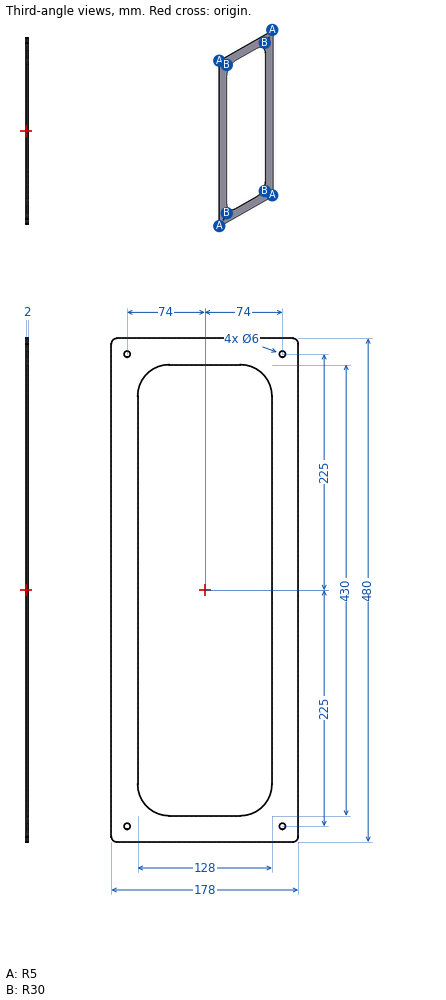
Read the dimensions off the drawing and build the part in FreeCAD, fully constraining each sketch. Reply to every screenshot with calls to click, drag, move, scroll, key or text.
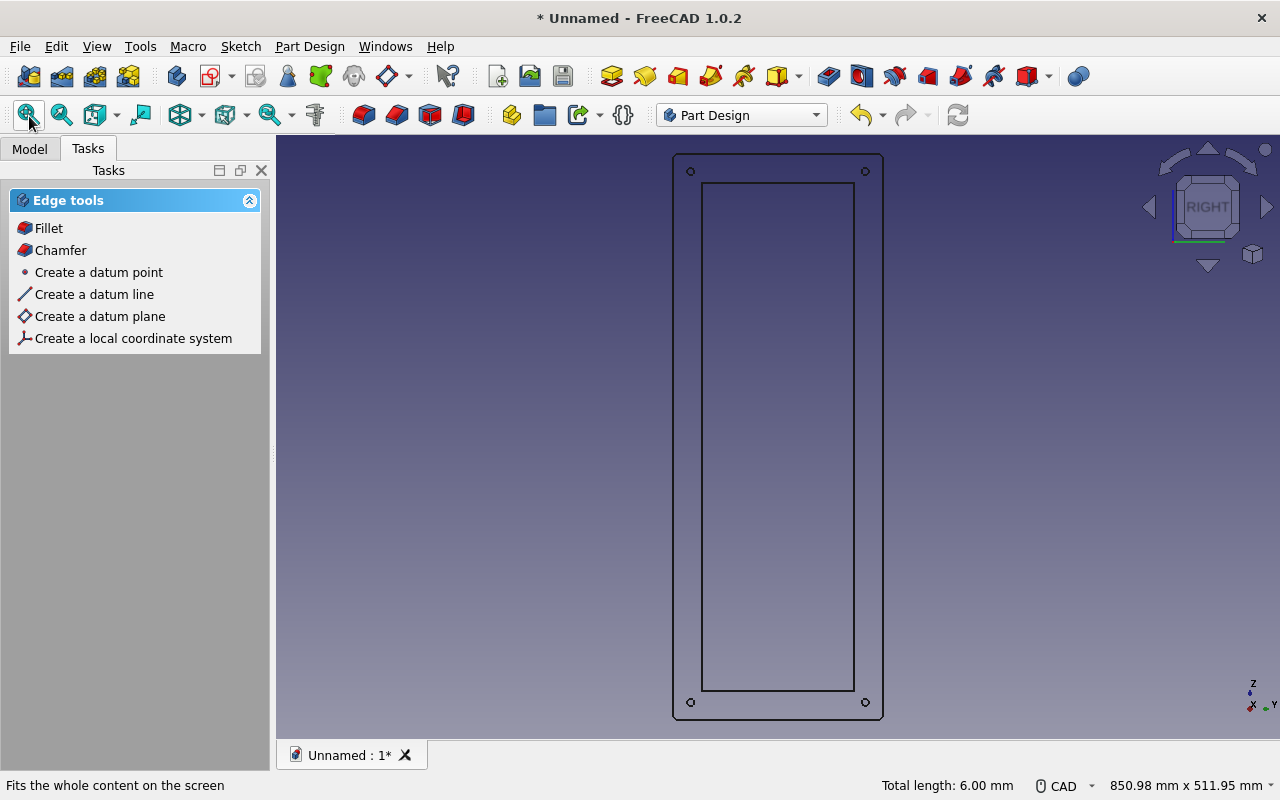
scroll(854, 690, up, 15)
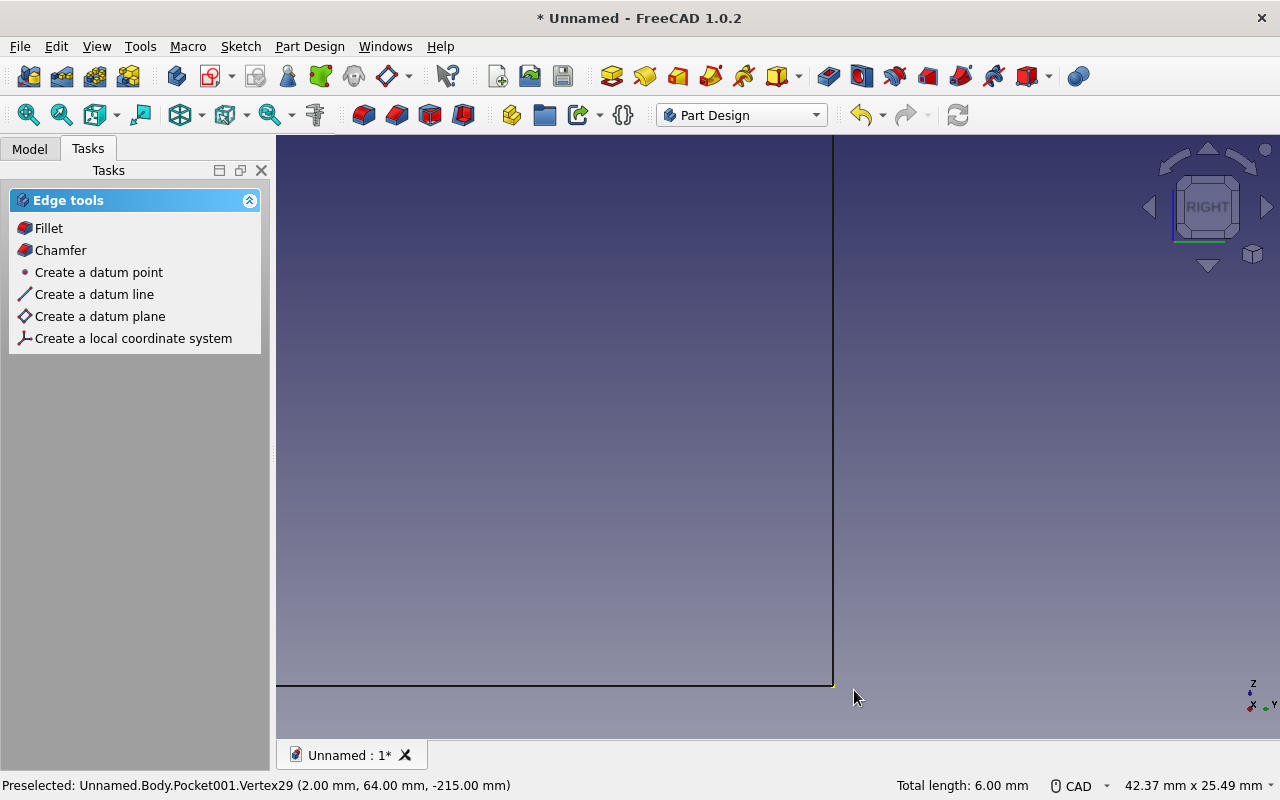
key(v)
key(f)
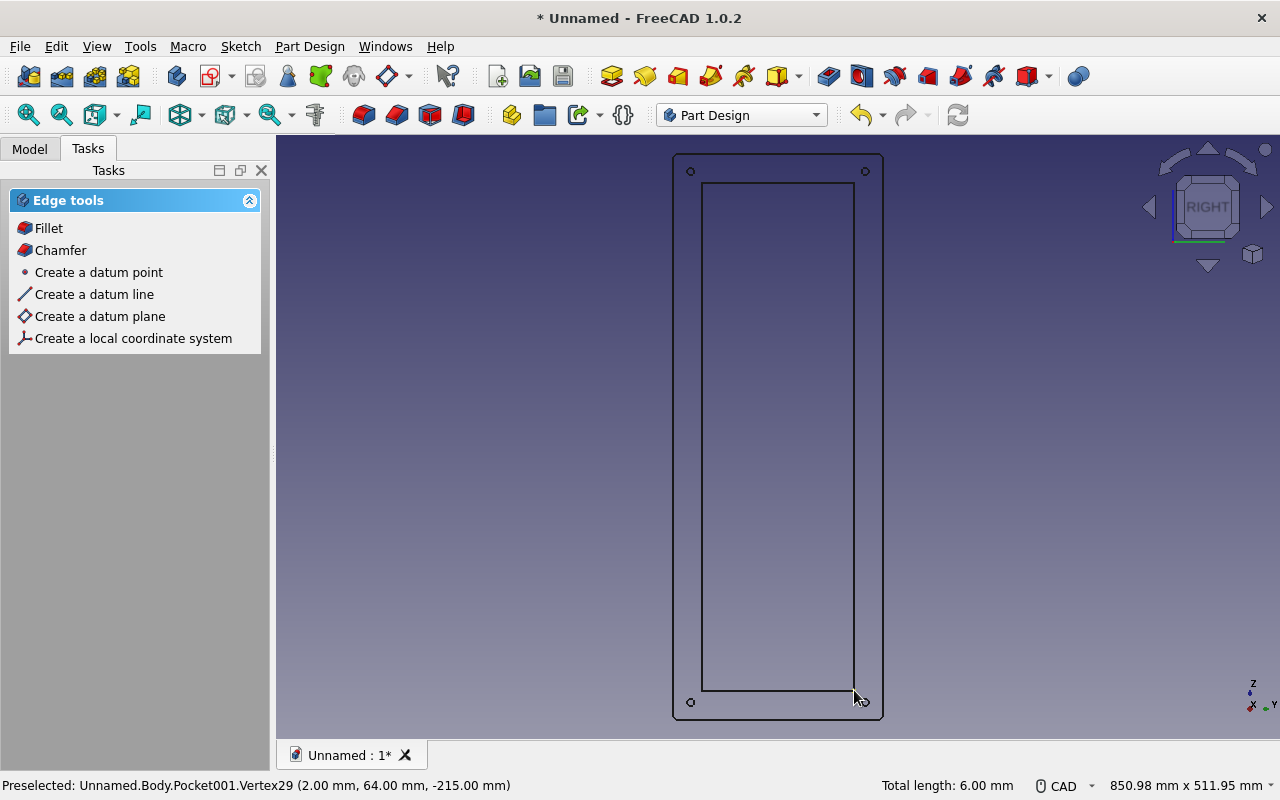
key(5)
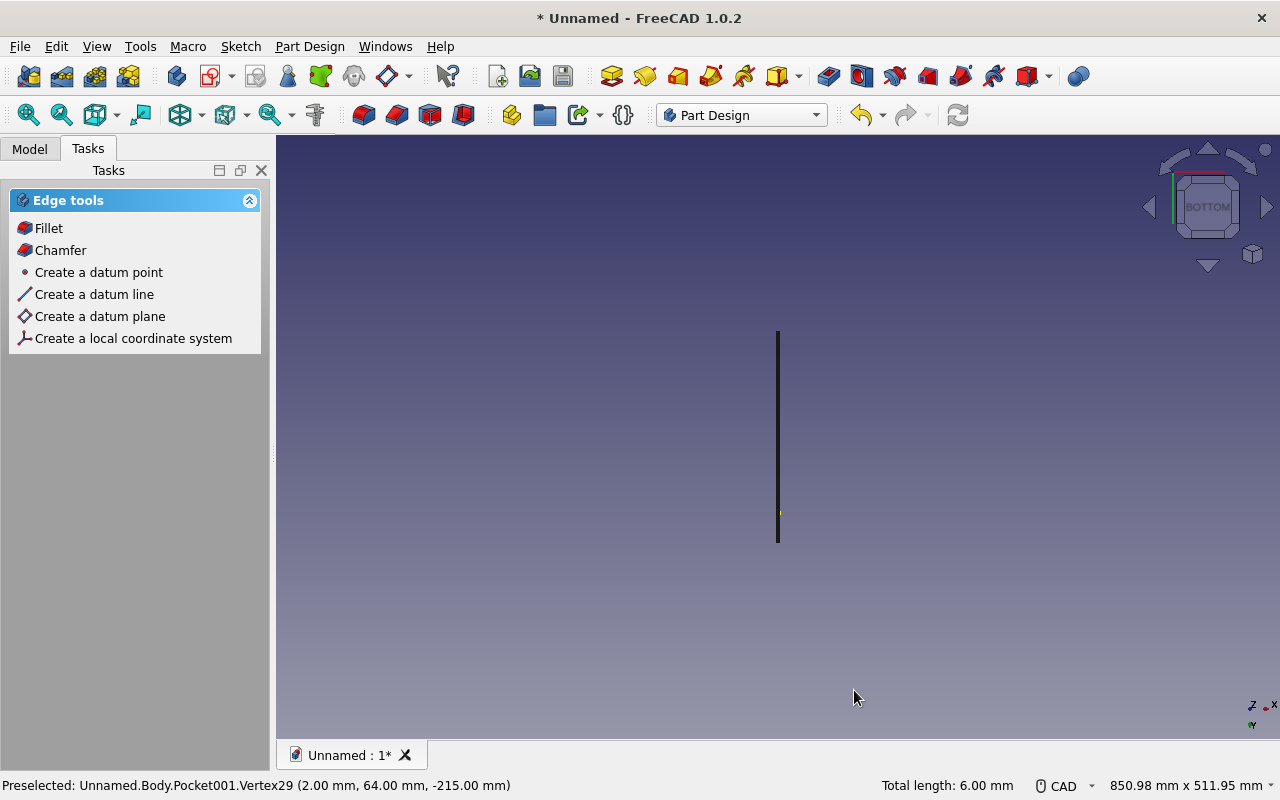
key(v)
key(f)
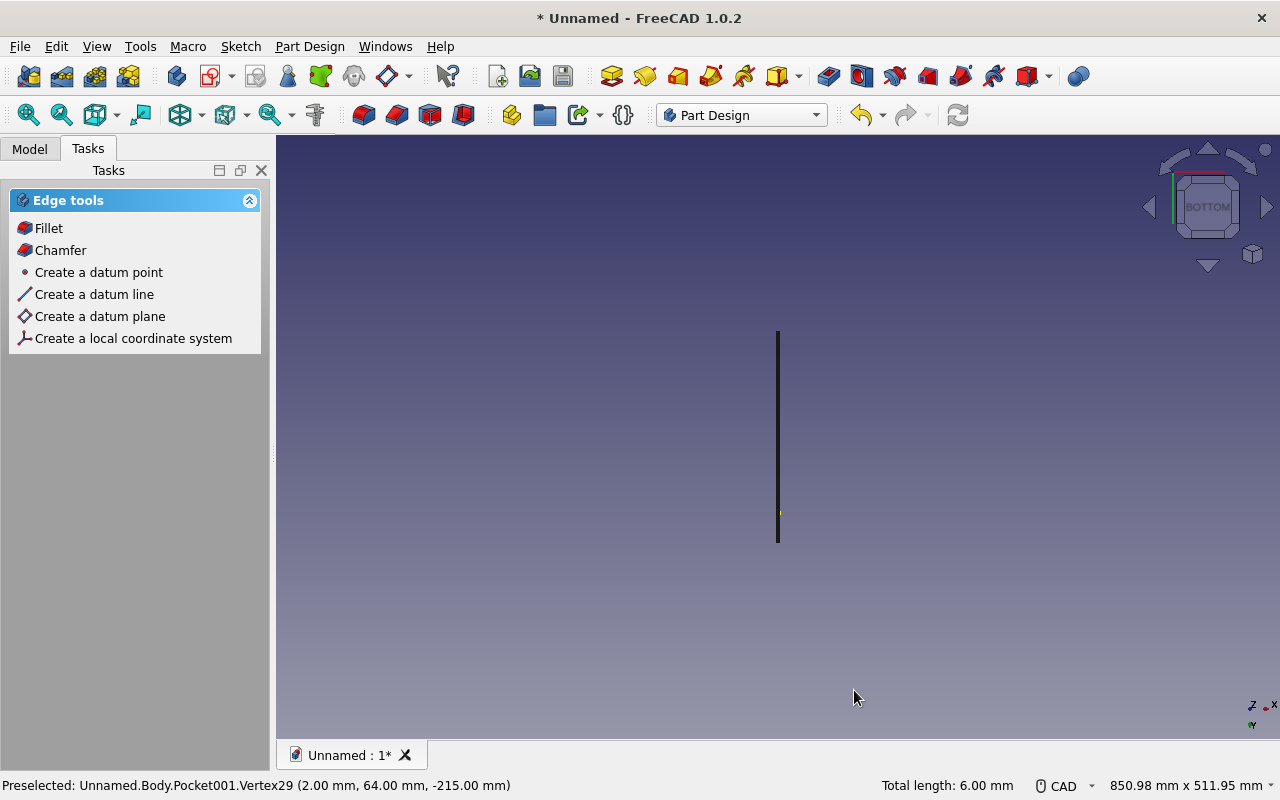
scroll(778, 512, up, 15)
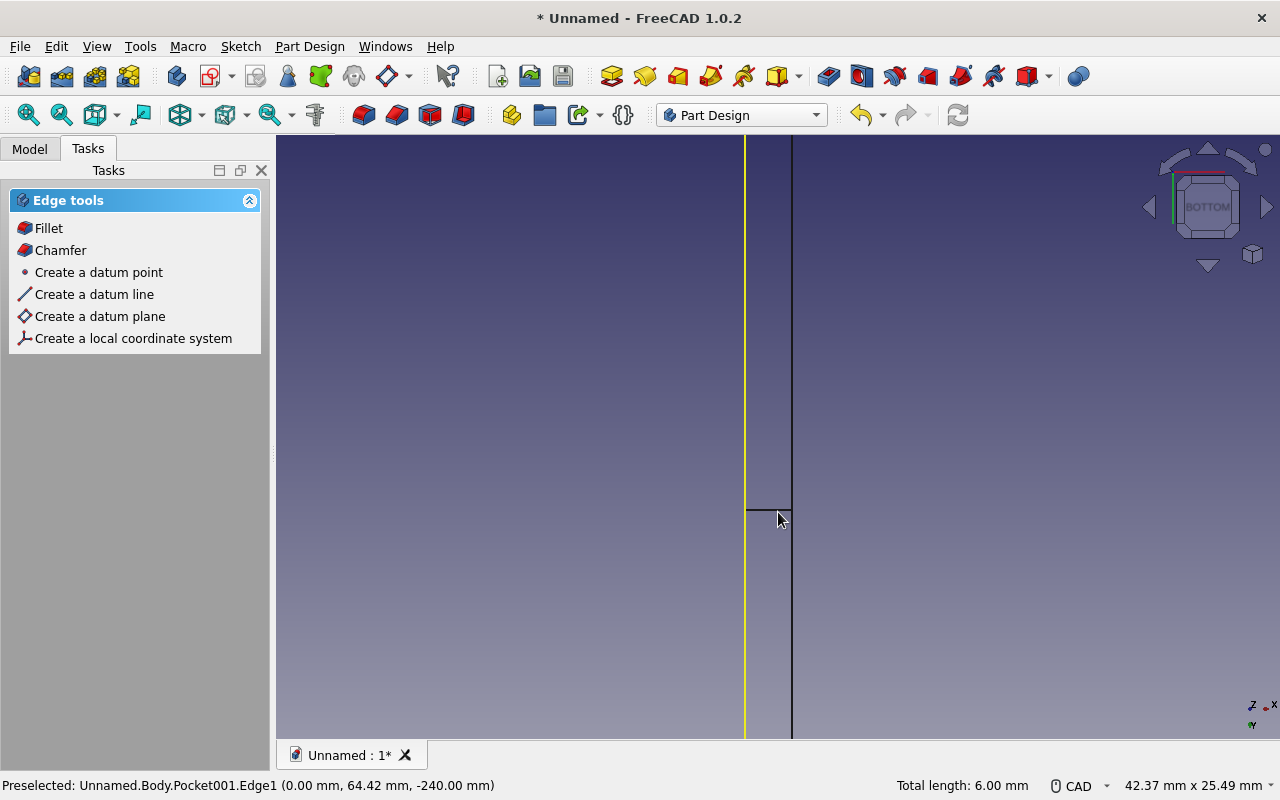
click(768, 509, ctrl)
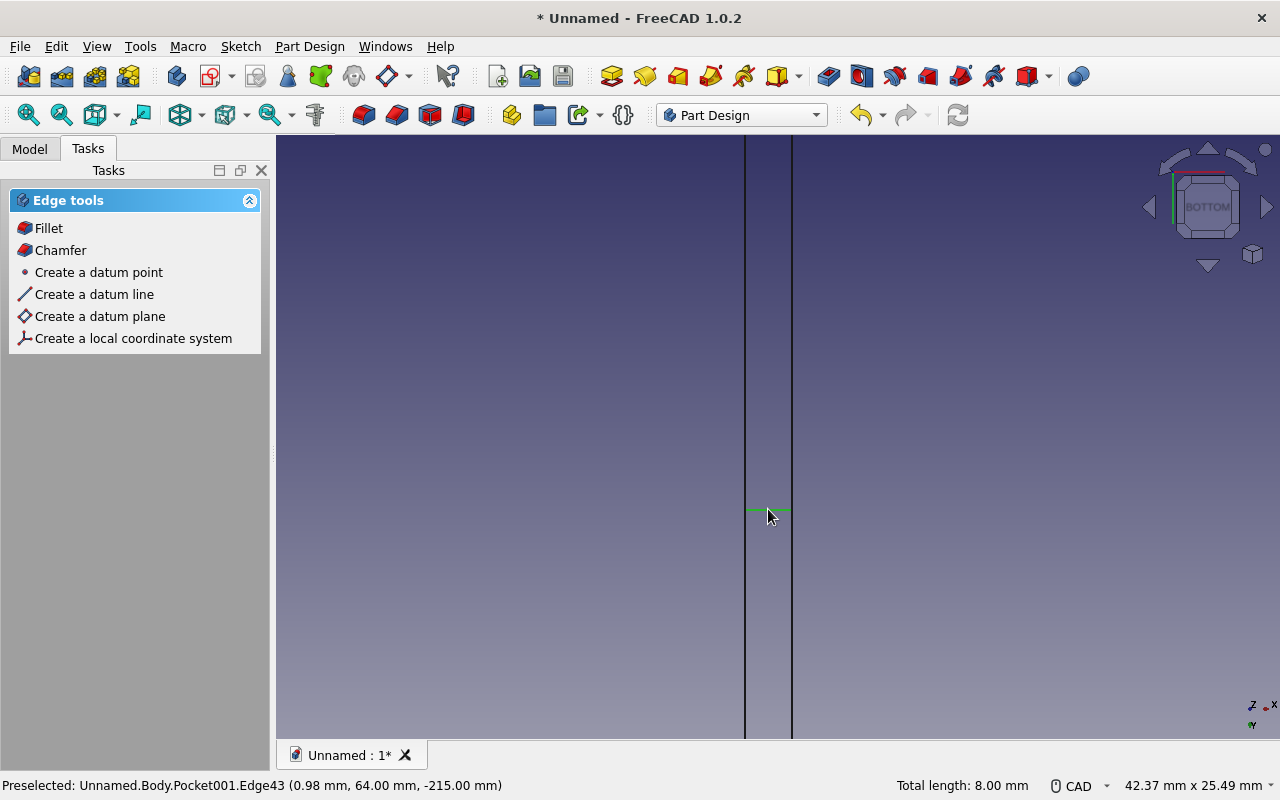
key(v)
key(1)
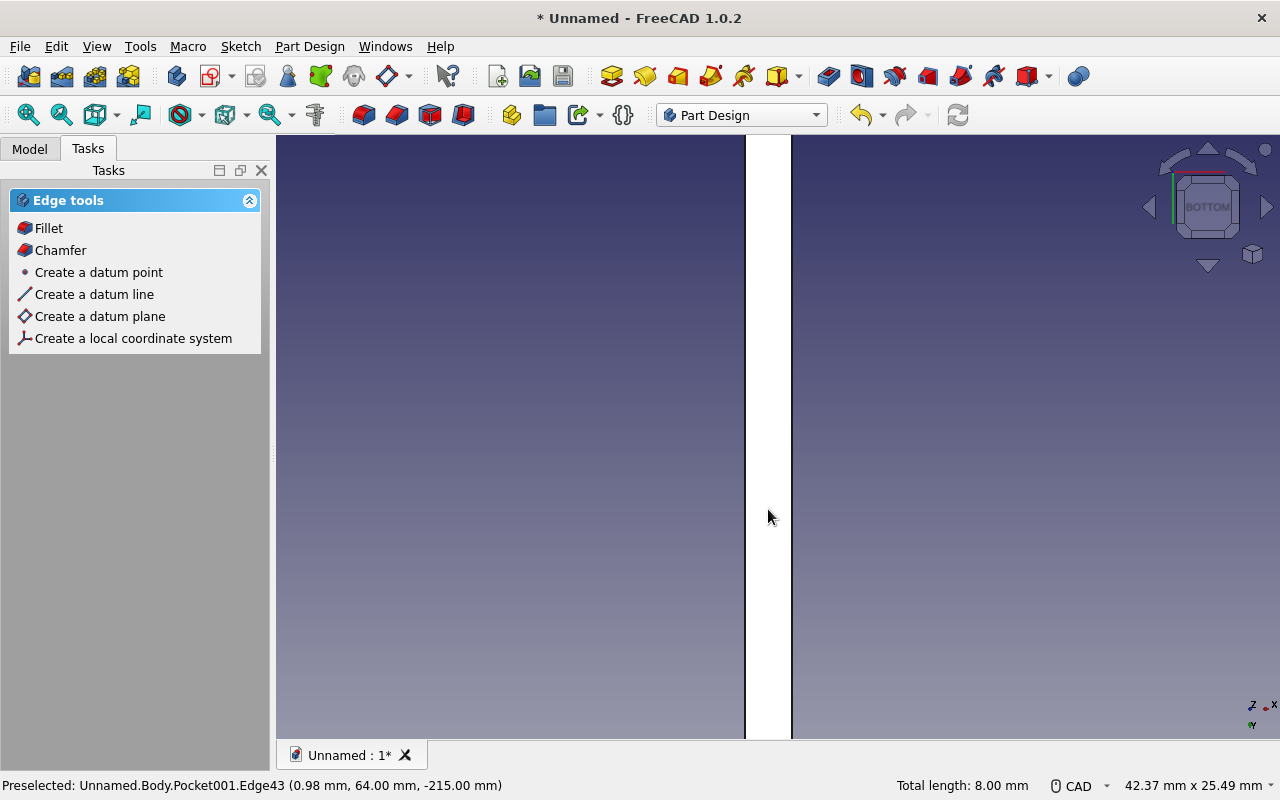
click(364, 116)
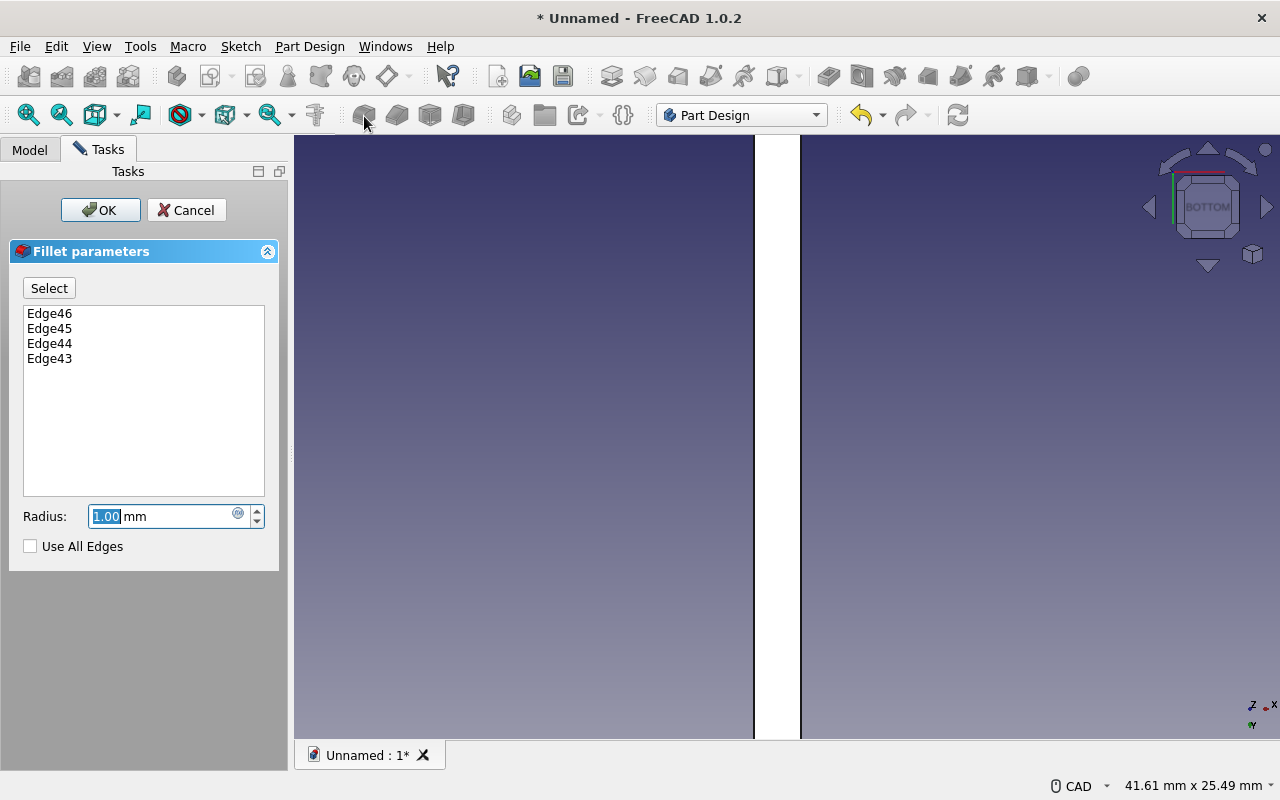
text(30)
key(Tab)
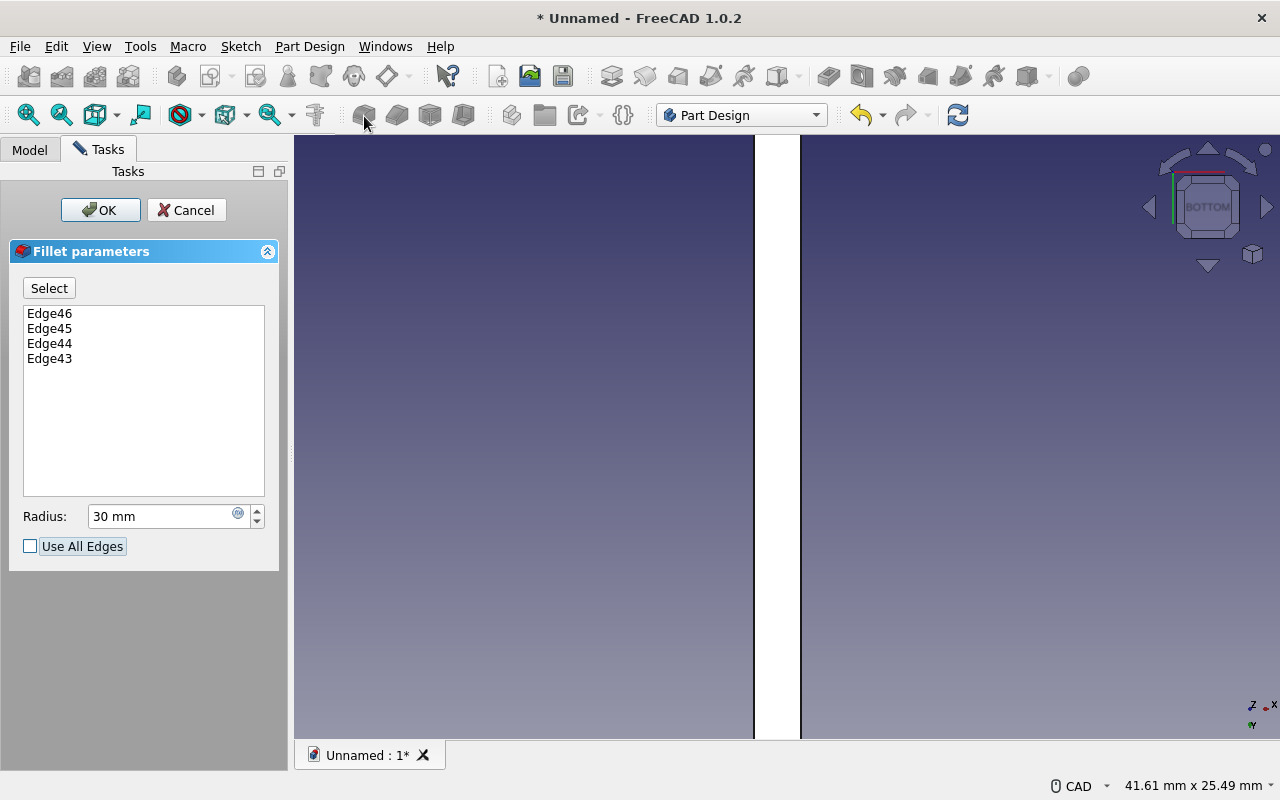
click(101, 210)